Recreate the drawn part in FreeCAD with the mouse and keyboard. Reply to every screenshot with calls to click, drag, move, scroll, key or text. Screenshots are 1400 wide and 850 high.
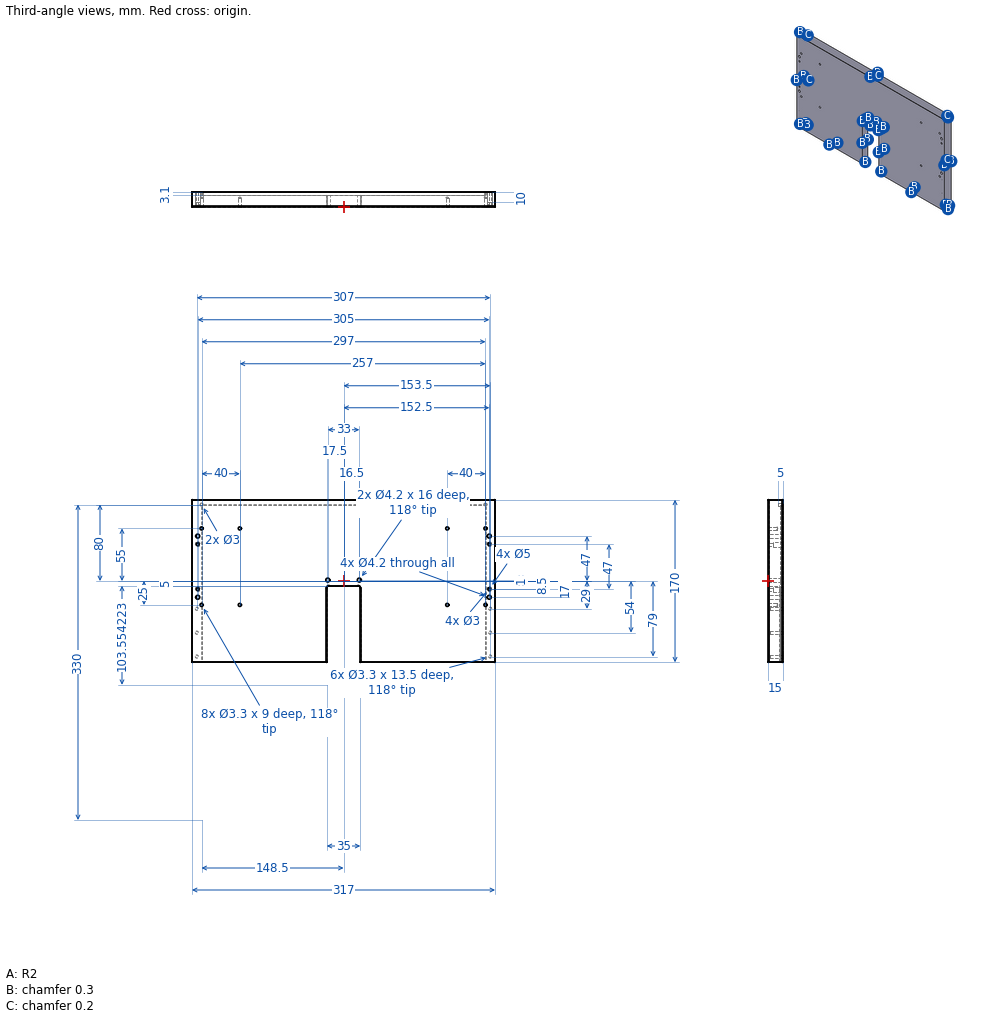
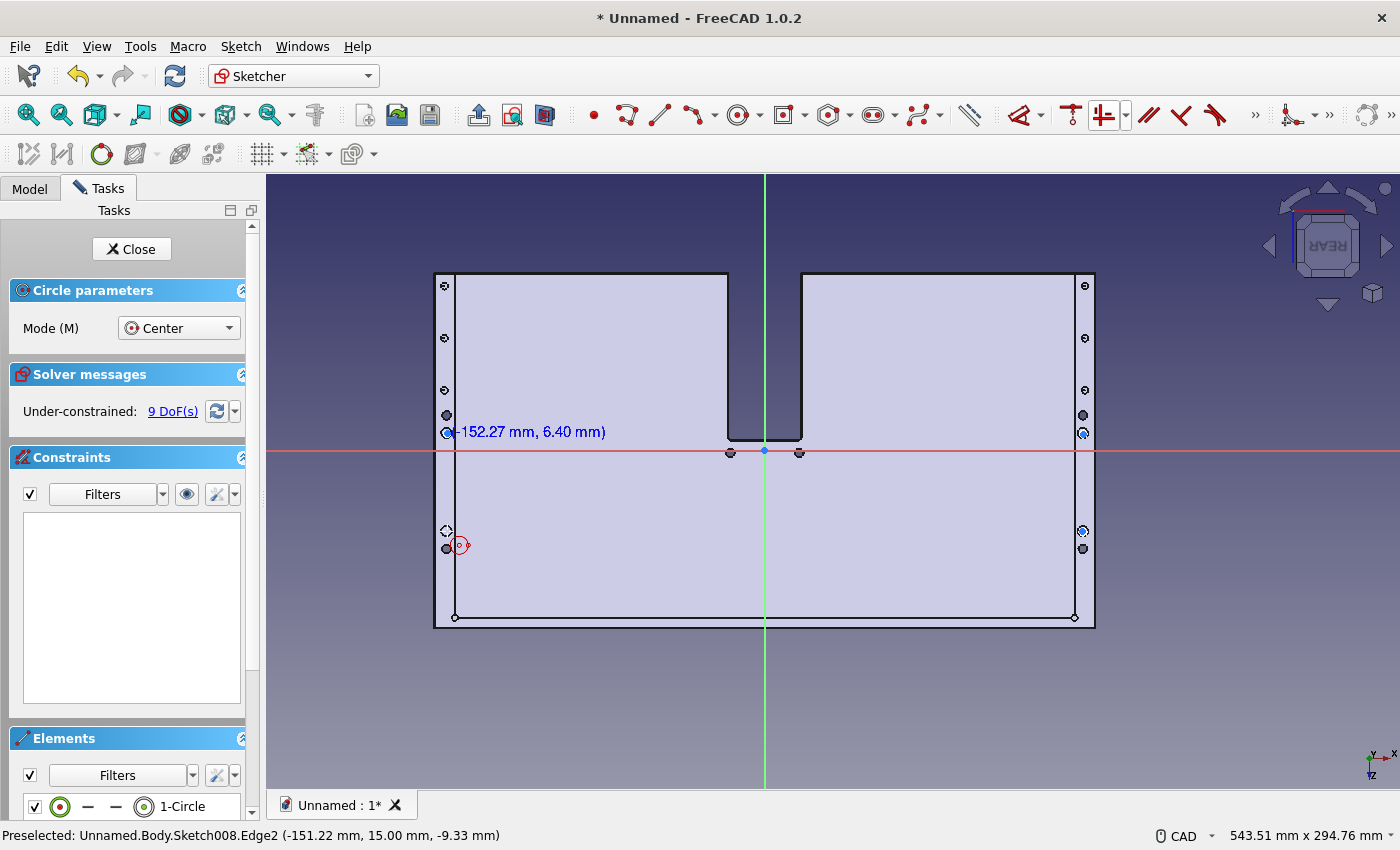
click(447, 531)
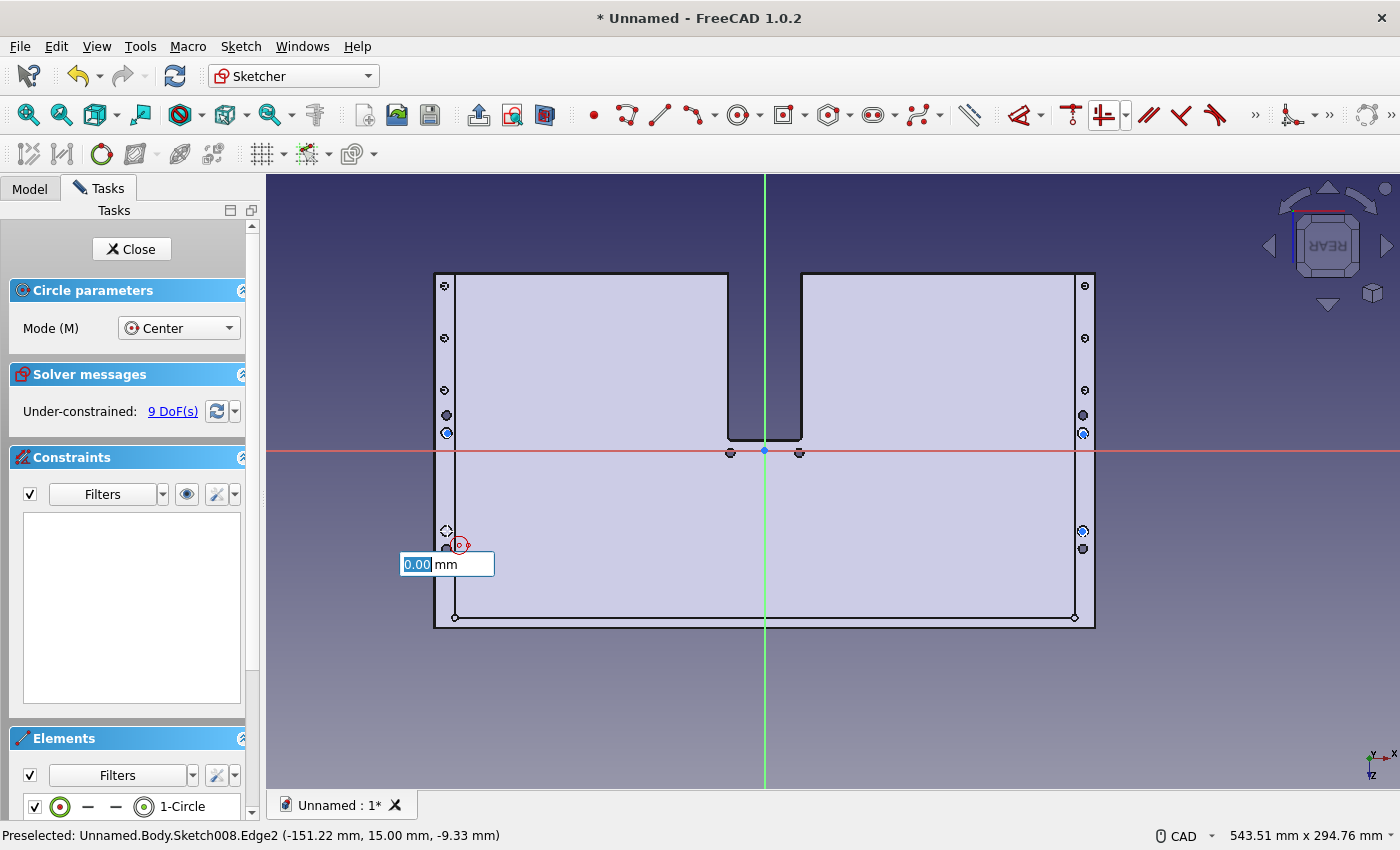
scroll(449, 529, up, 9)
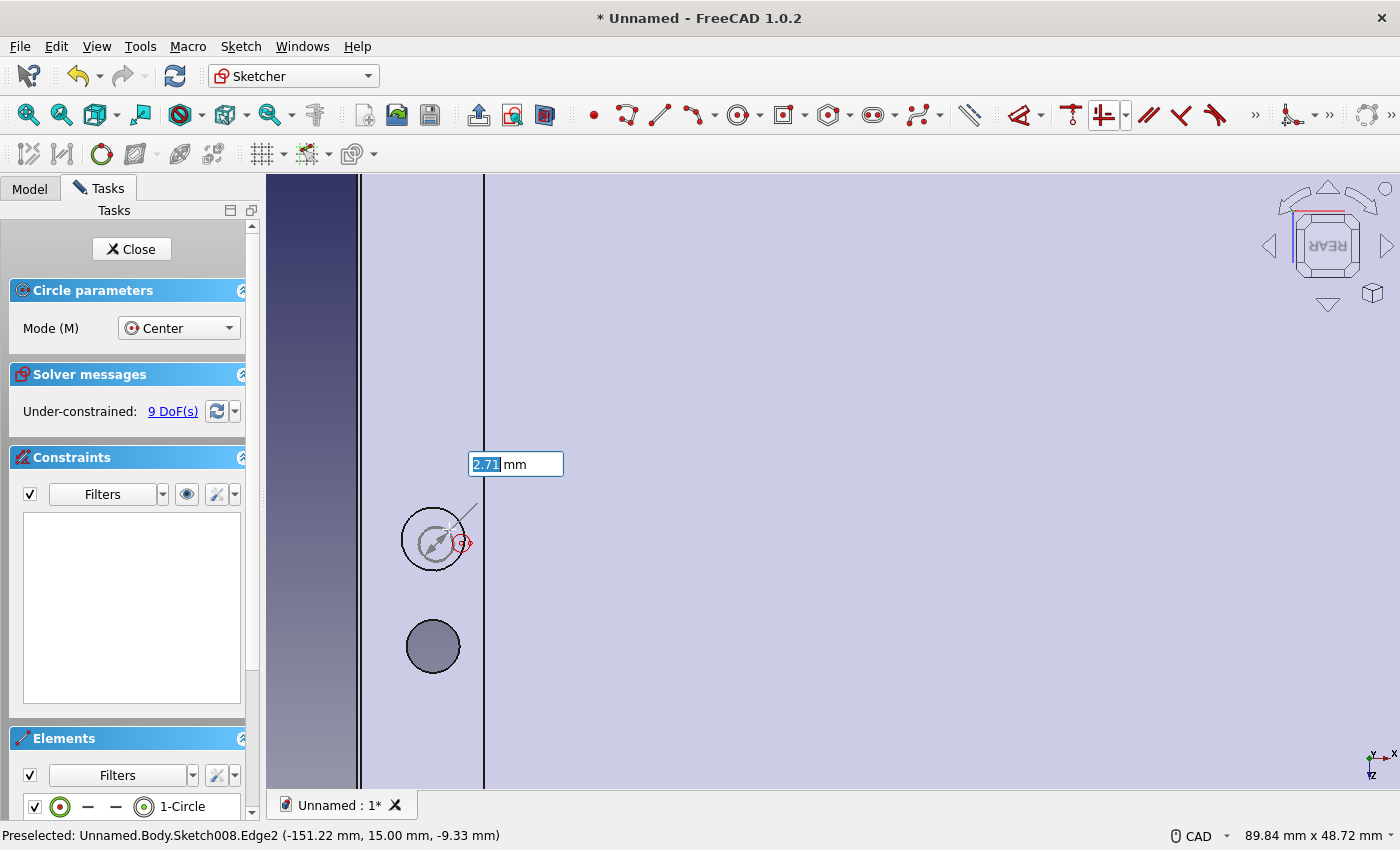
click(447, 526)
key(Escape)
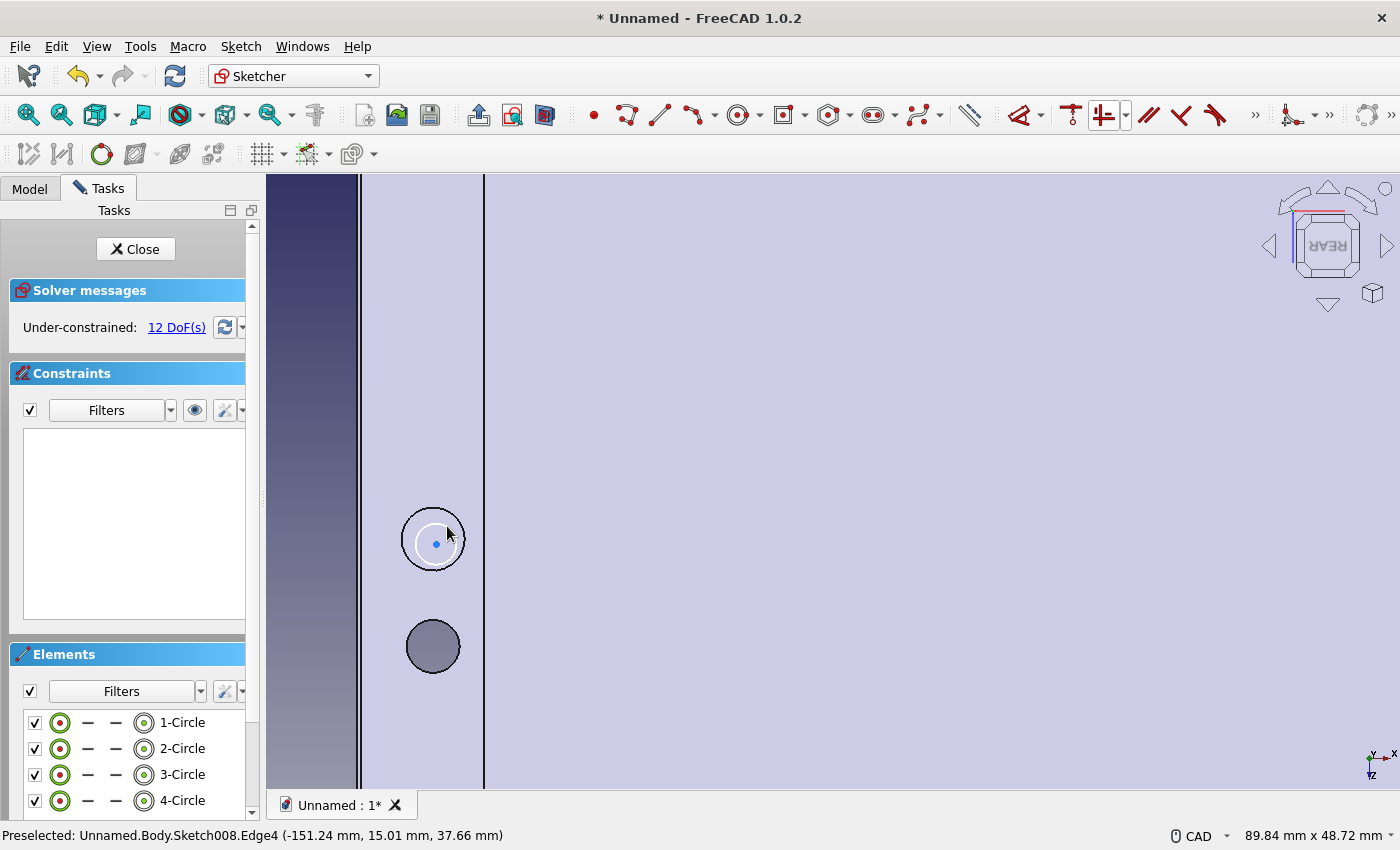
scroll(449, 529, down, 9)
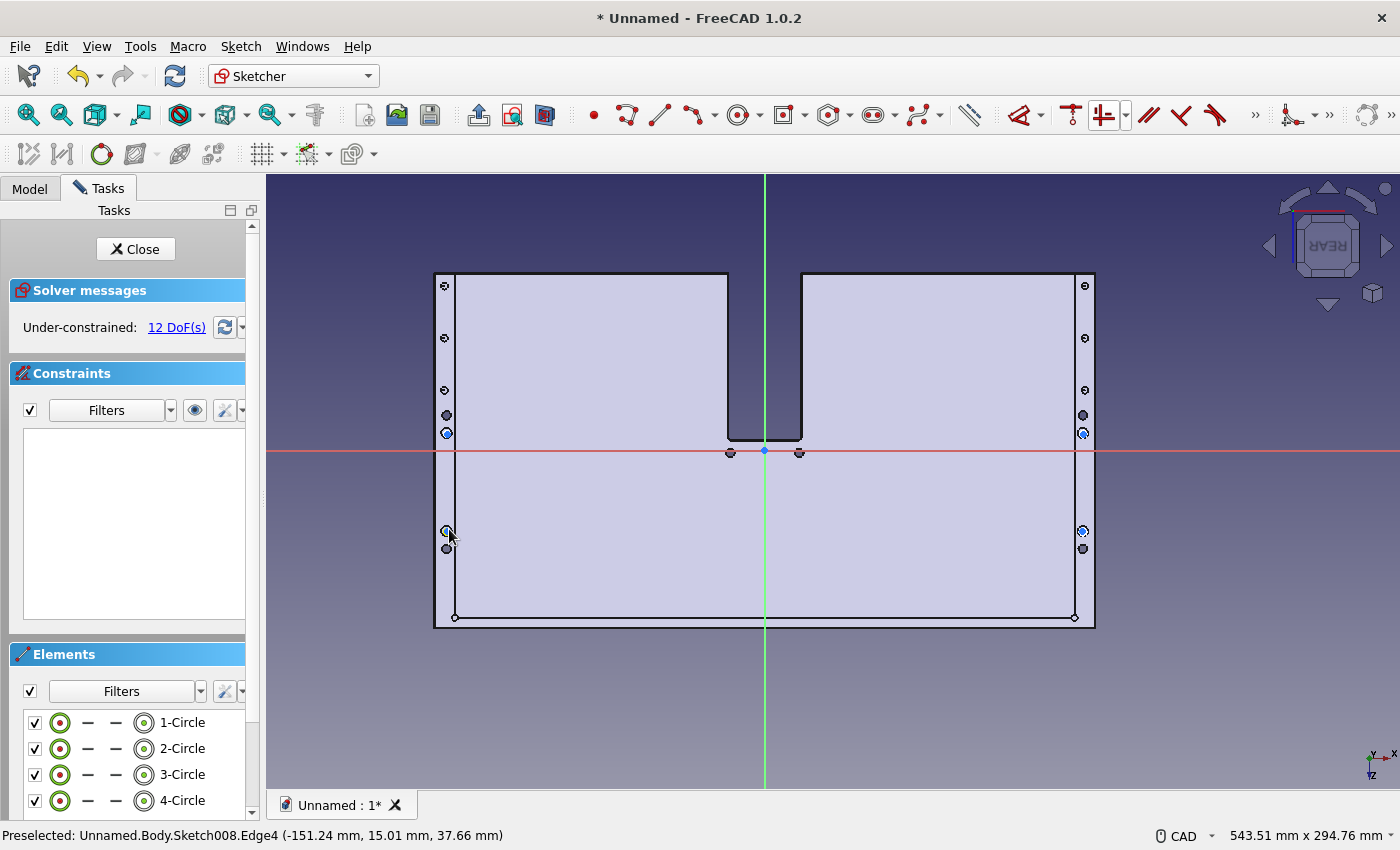
scroll(1086, 431, up, 7)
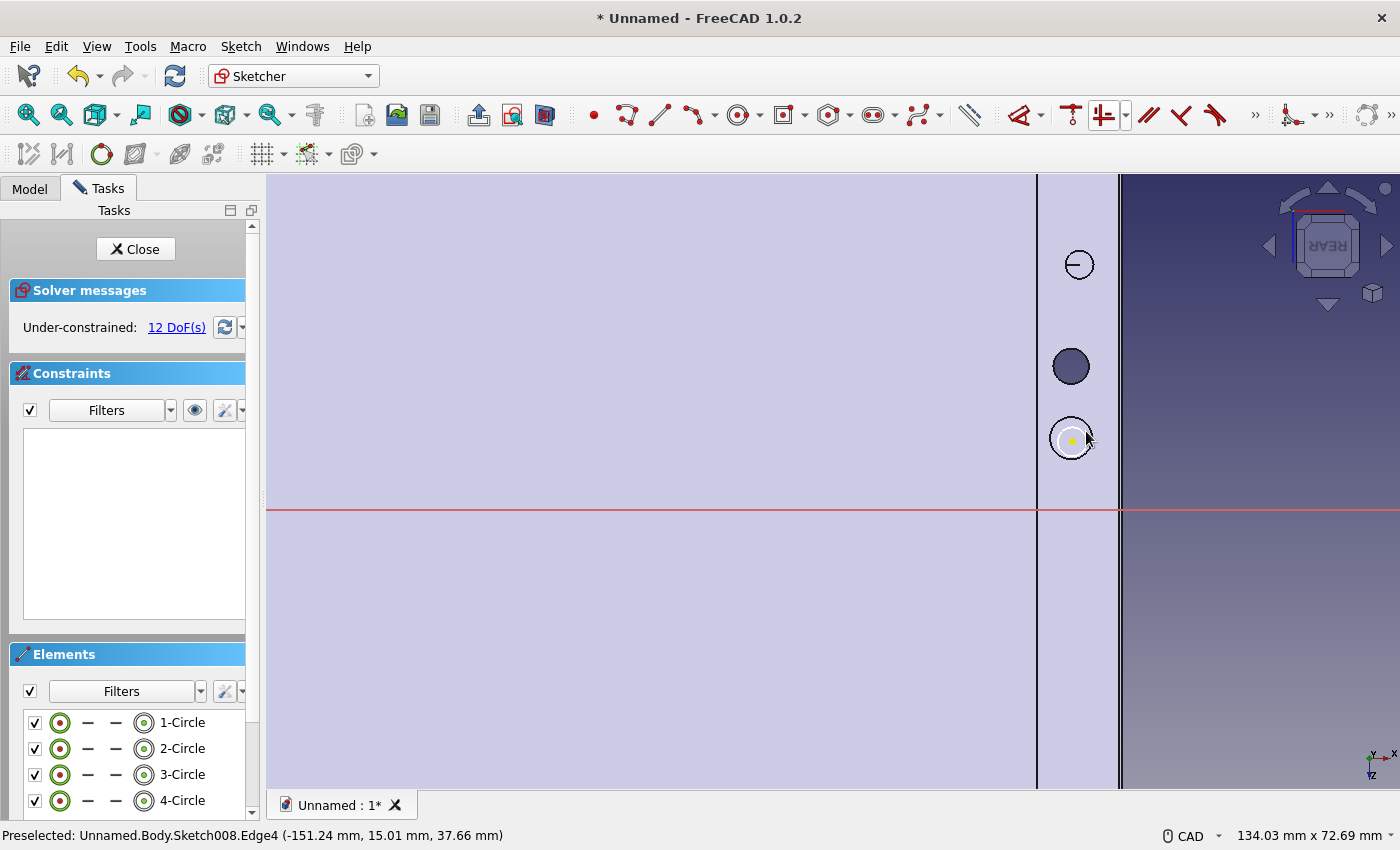
click(1082, 432)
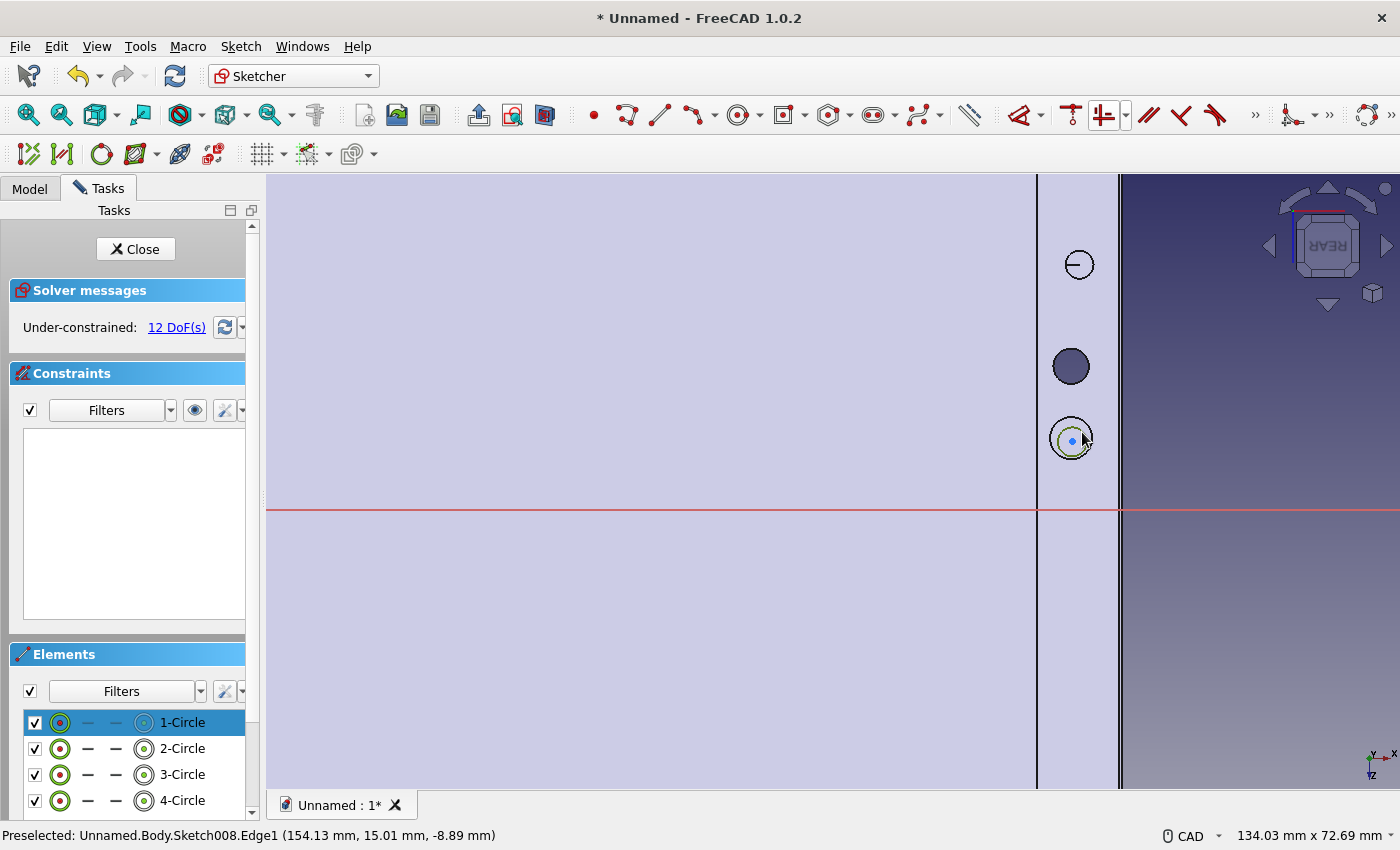
scroll(1086, 431, down, 7)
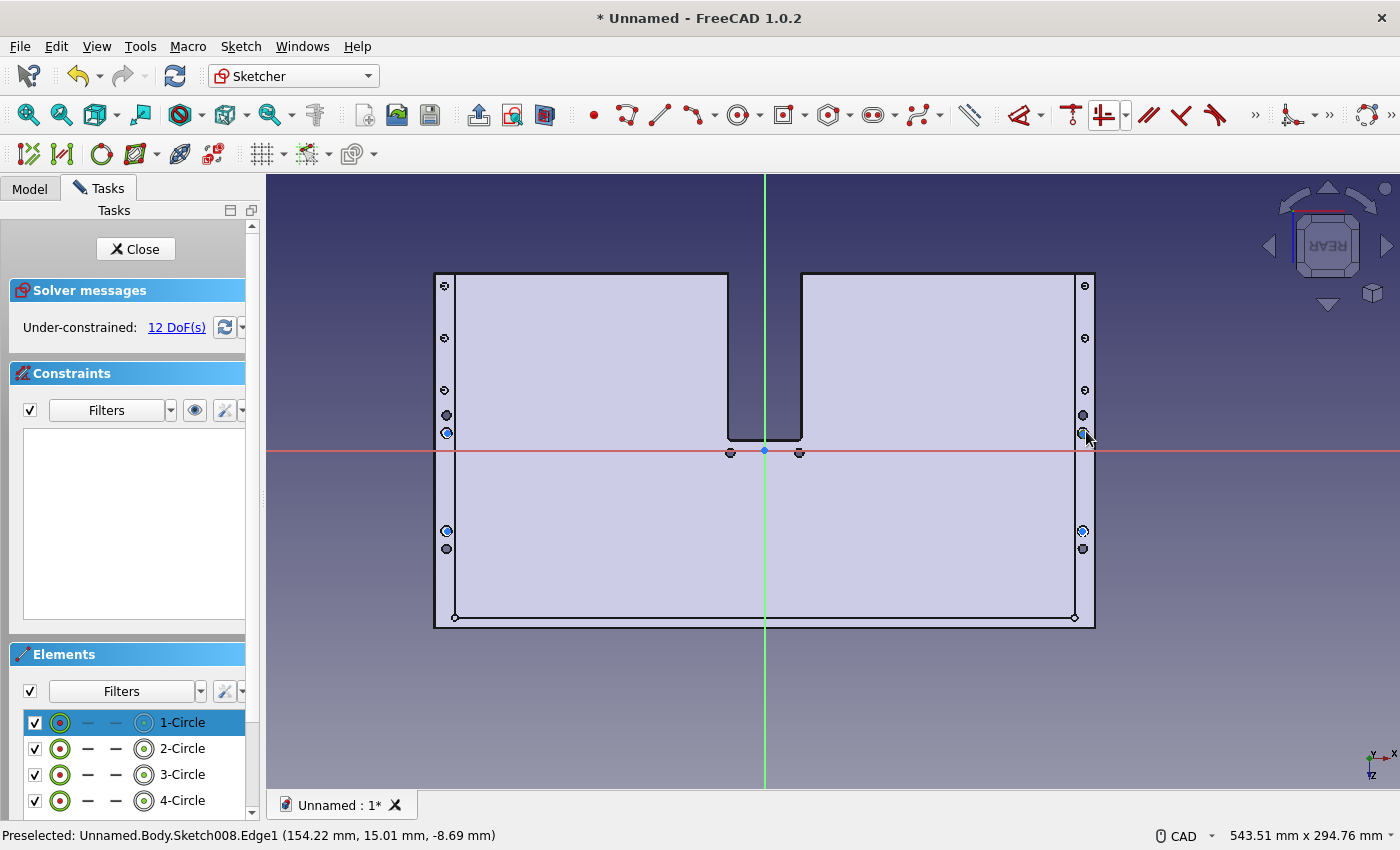
scroll(1085, 529, up, 7)